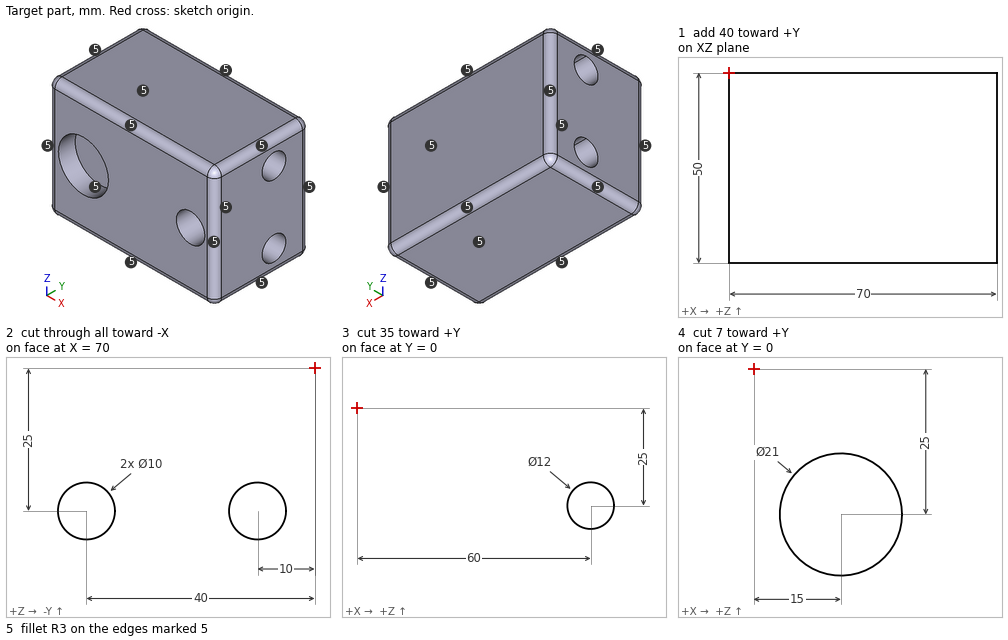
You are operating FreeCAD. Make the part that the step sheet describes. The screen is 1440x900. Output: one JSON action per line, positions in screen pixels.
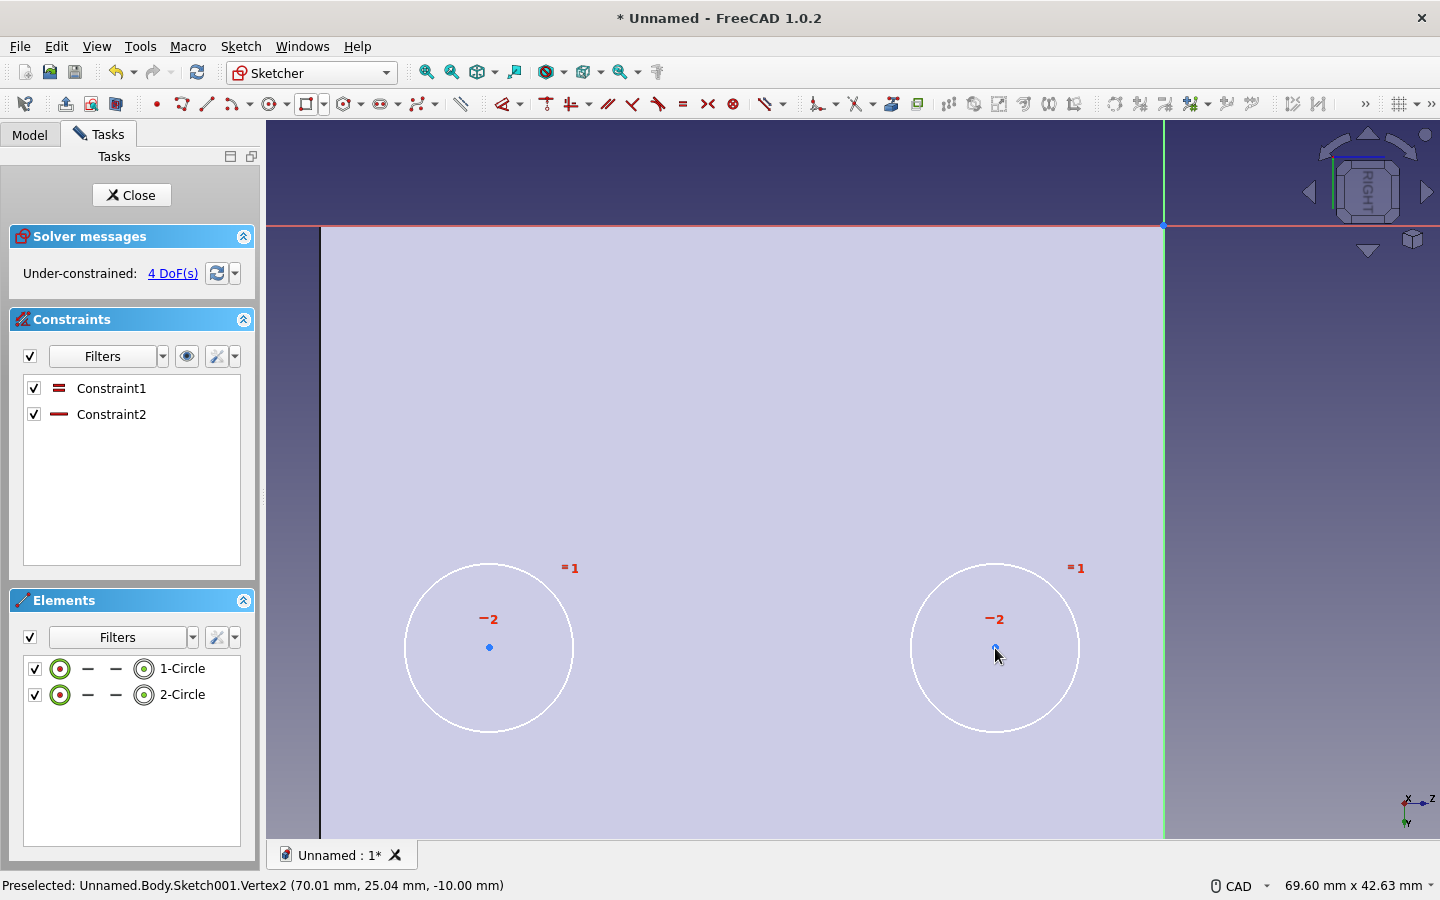
{"action": "left_click", "coordinate": [548, 588]}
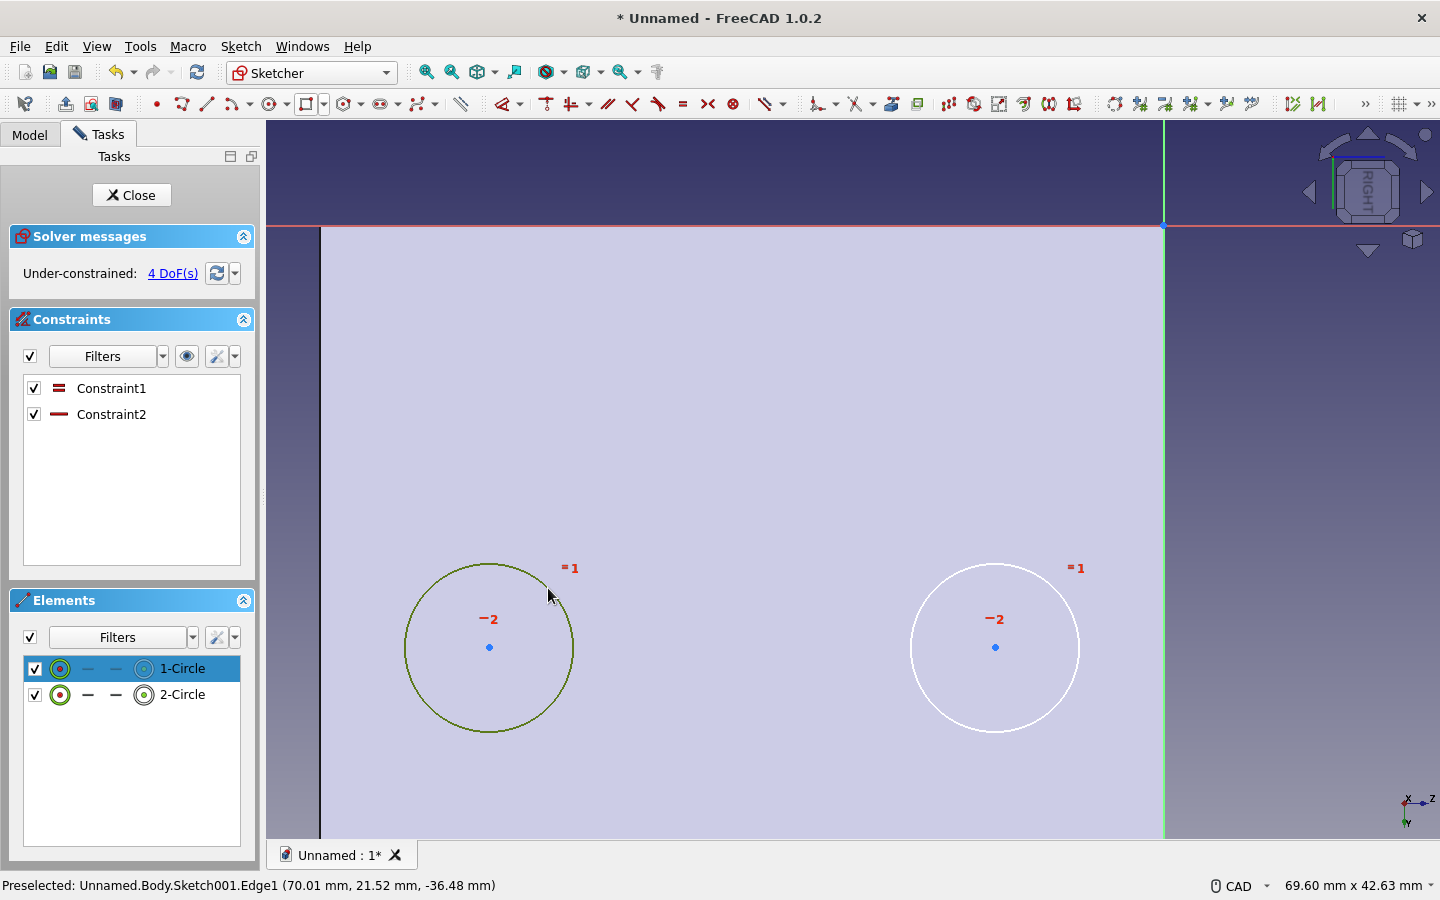
{"action": "key", "text": "k o"}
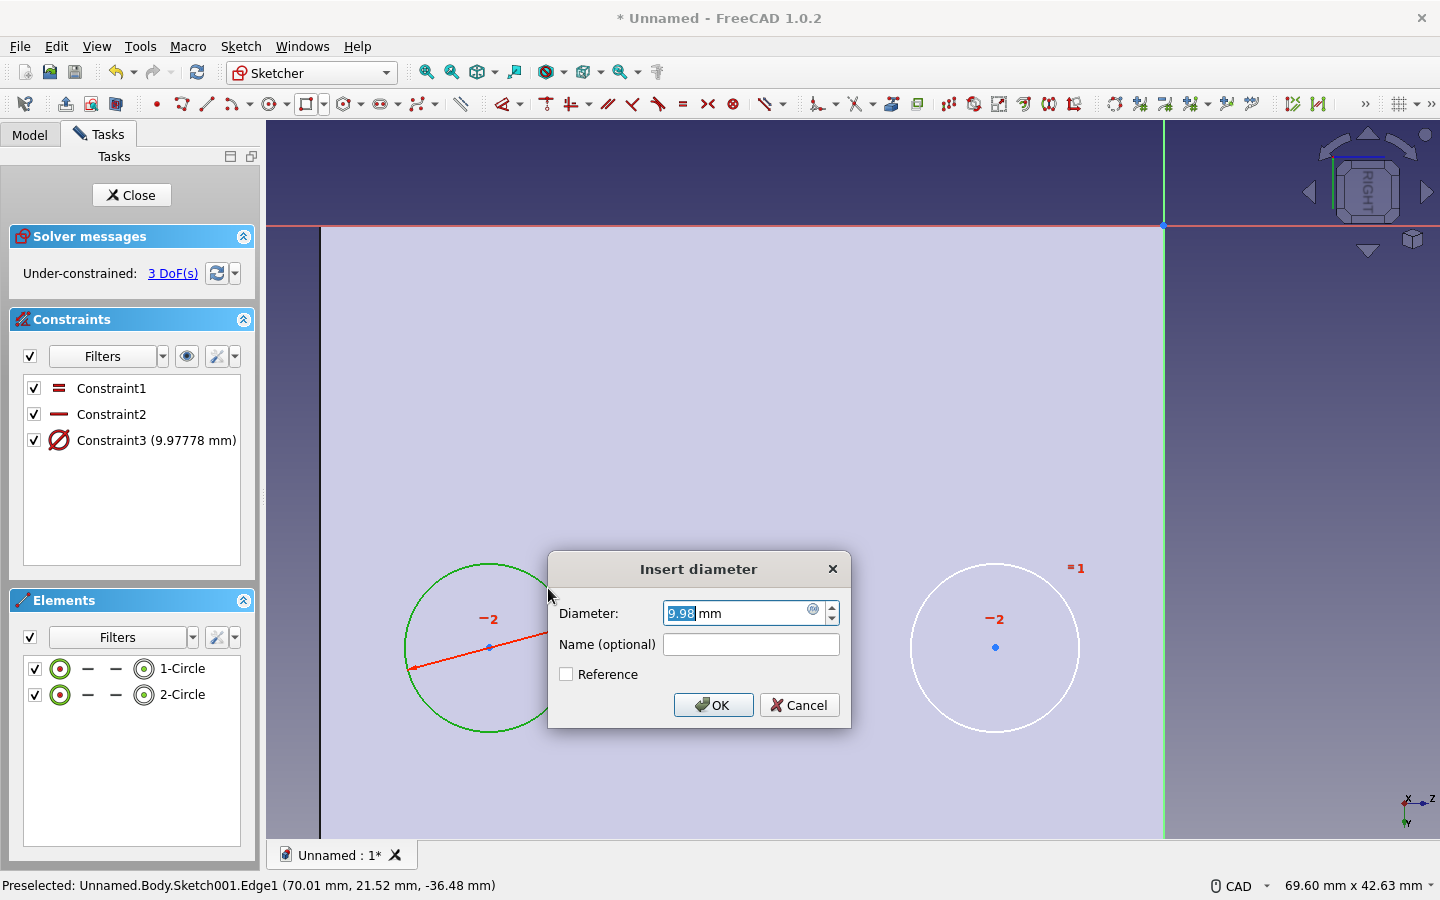
{"action": "type", "text": "10"}
{"action": "key", "text": "Return"}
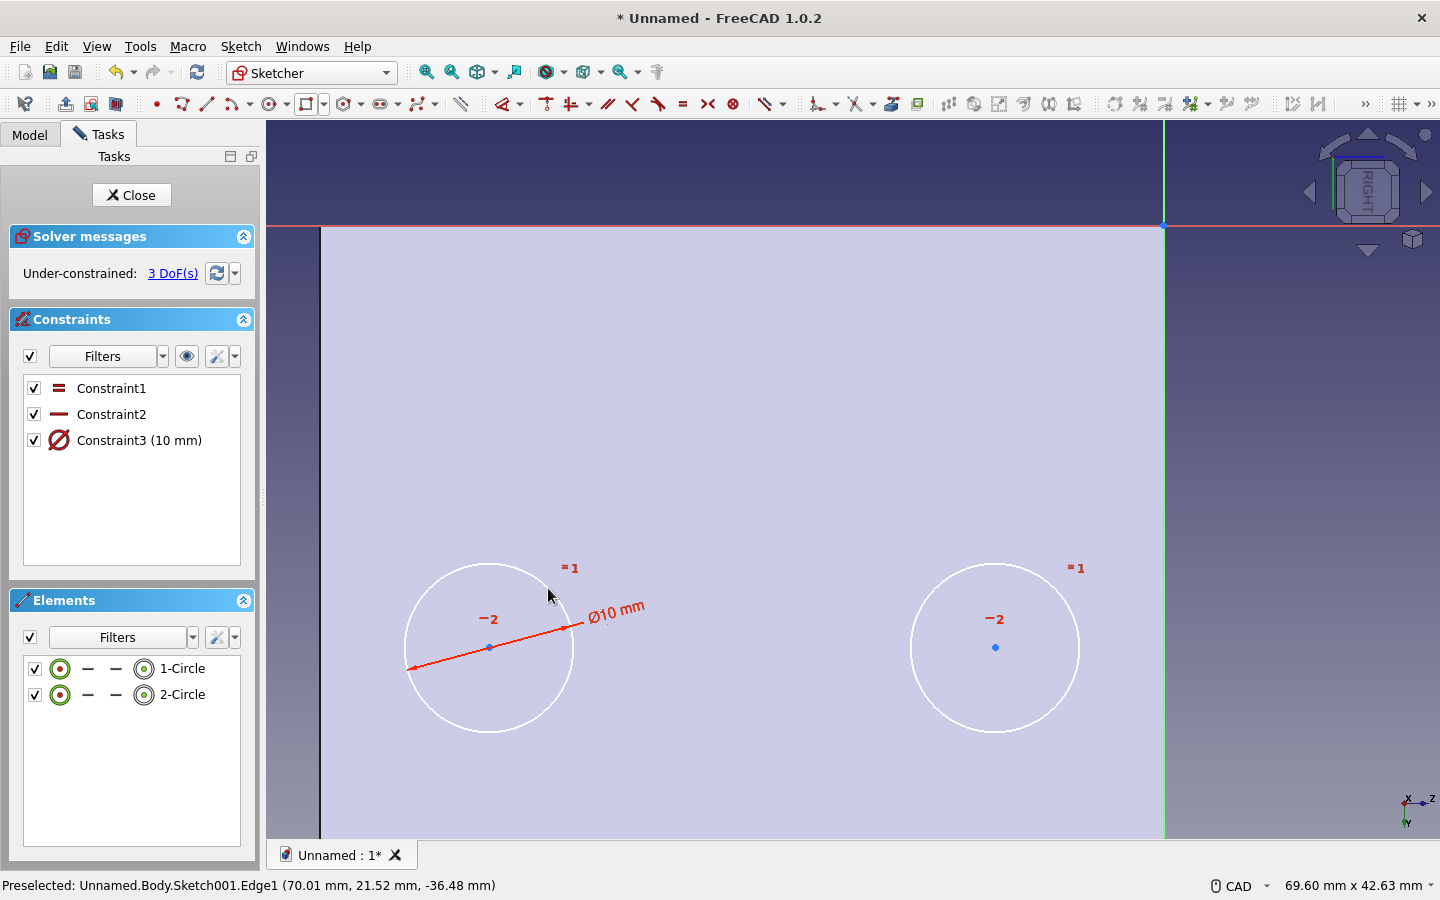
{"action": "left_click", "coordinate": [489, 648]}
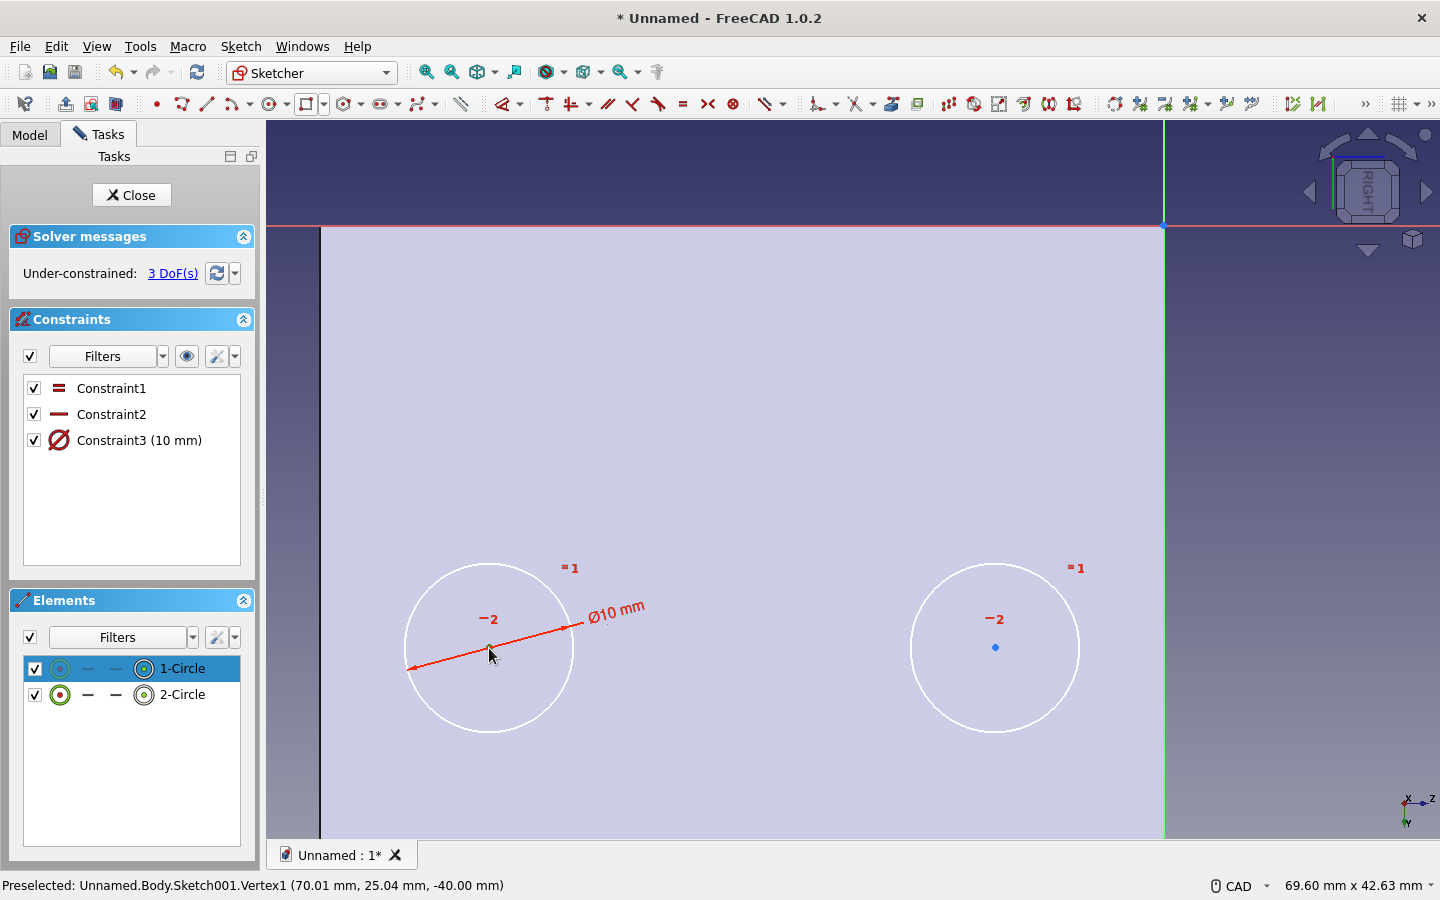
{"action": "key", "text": "l"}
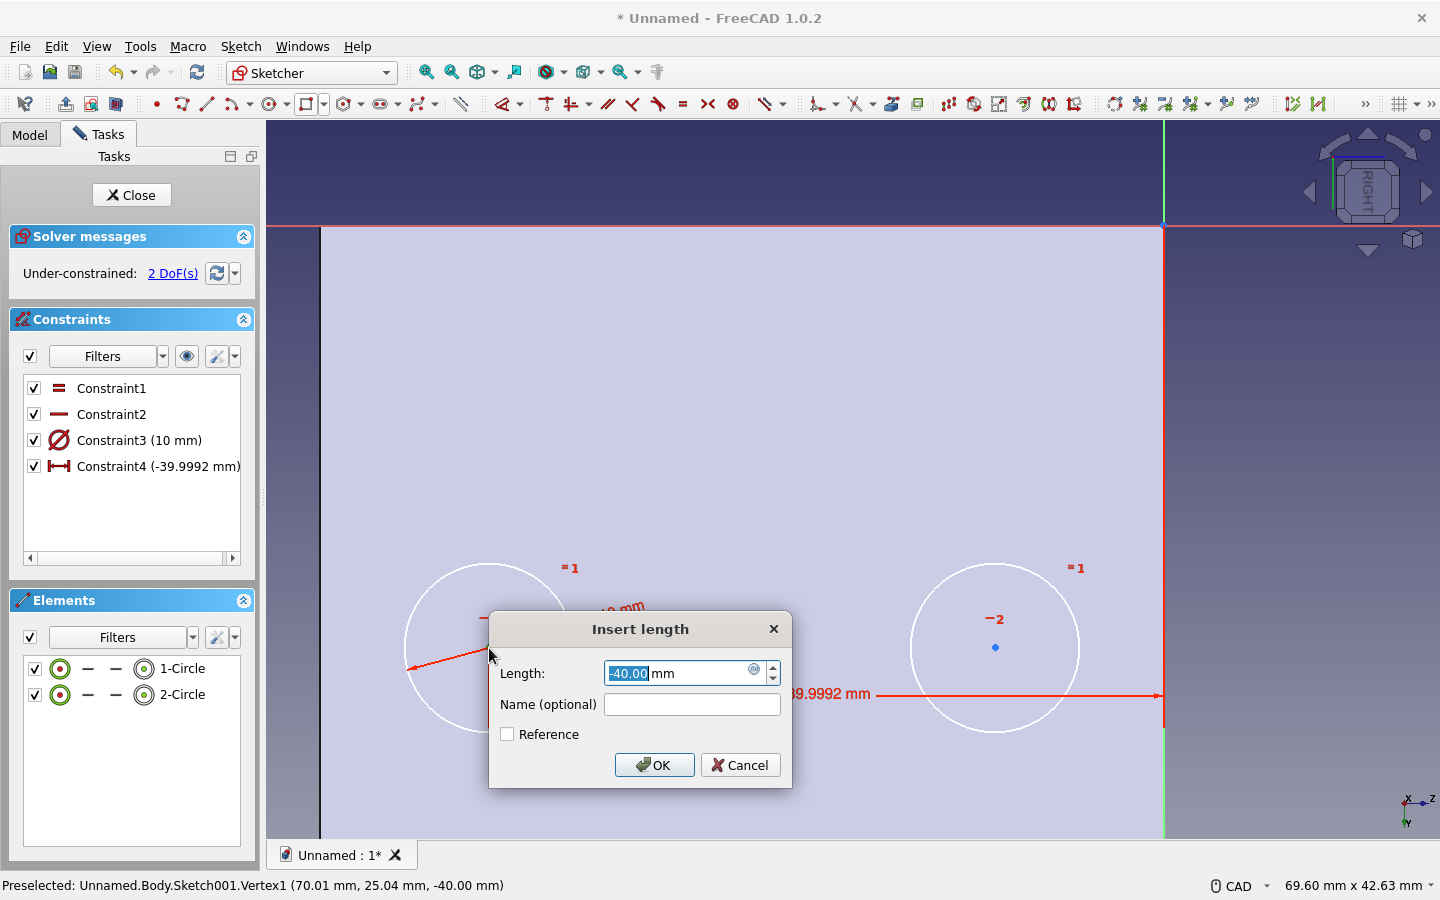
{"action": "type", "text": "-40"}
{"action": "key", "text": "Return"}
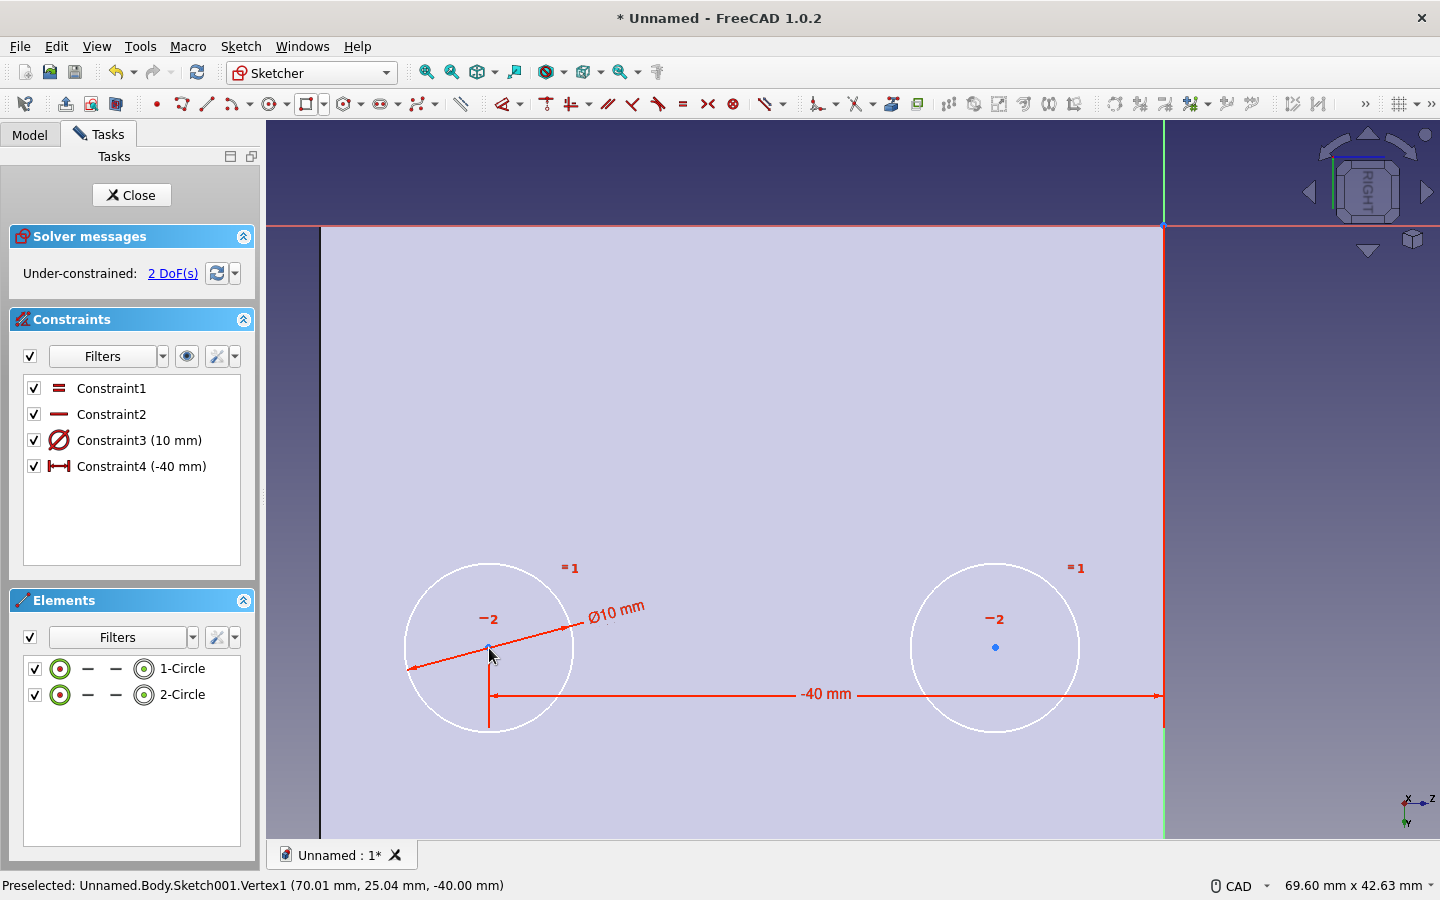
{"action": "left_click", "coordinate": [489, 648]}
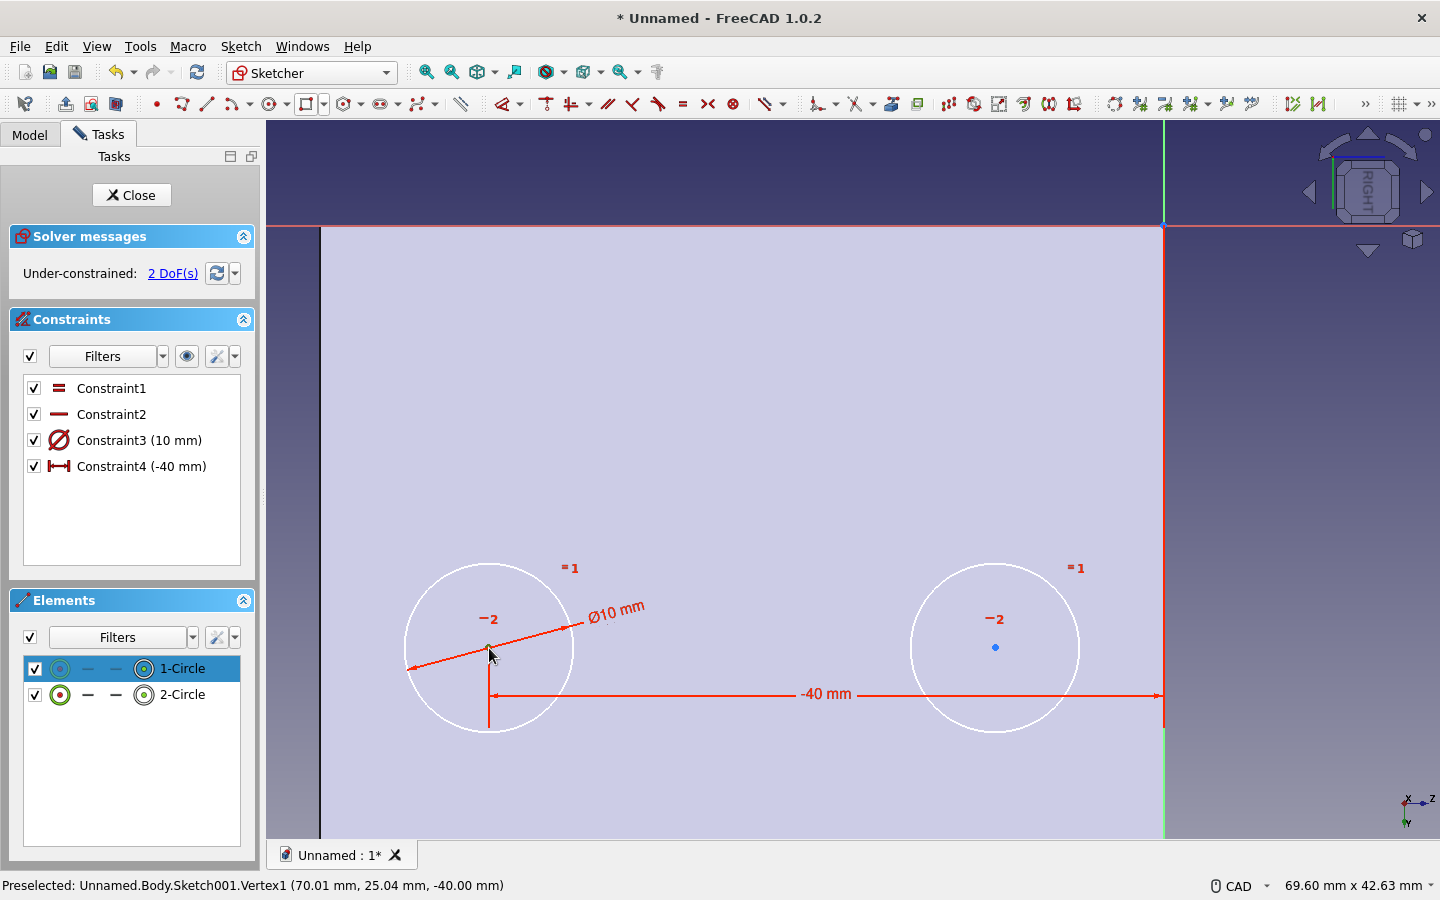
{"action": "key", "text": "i"}